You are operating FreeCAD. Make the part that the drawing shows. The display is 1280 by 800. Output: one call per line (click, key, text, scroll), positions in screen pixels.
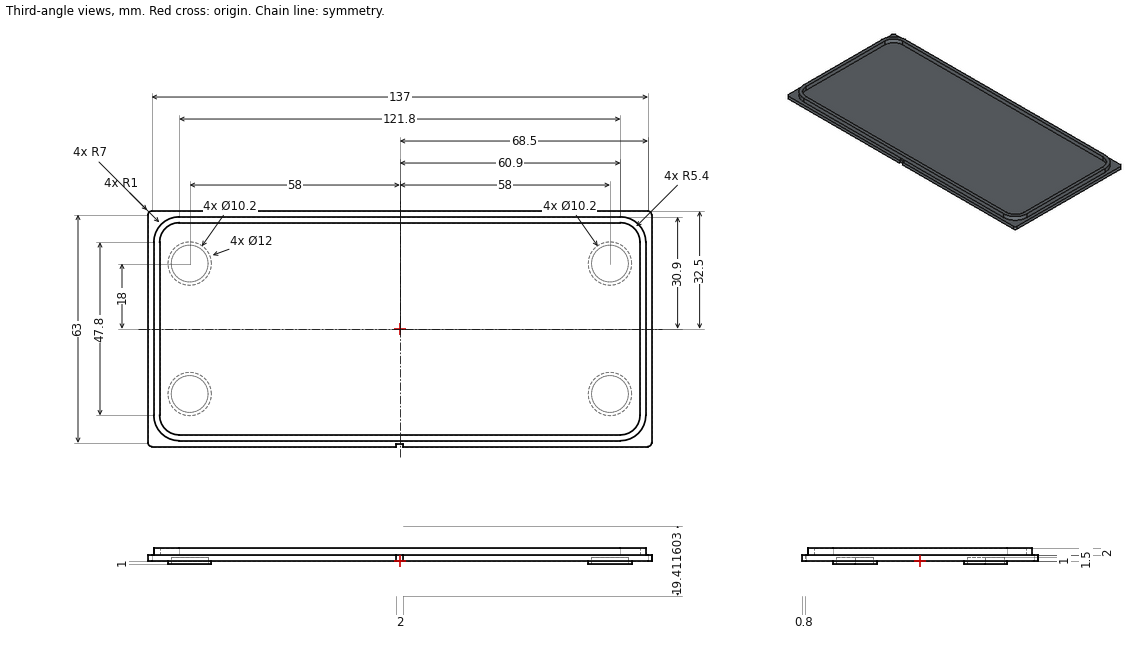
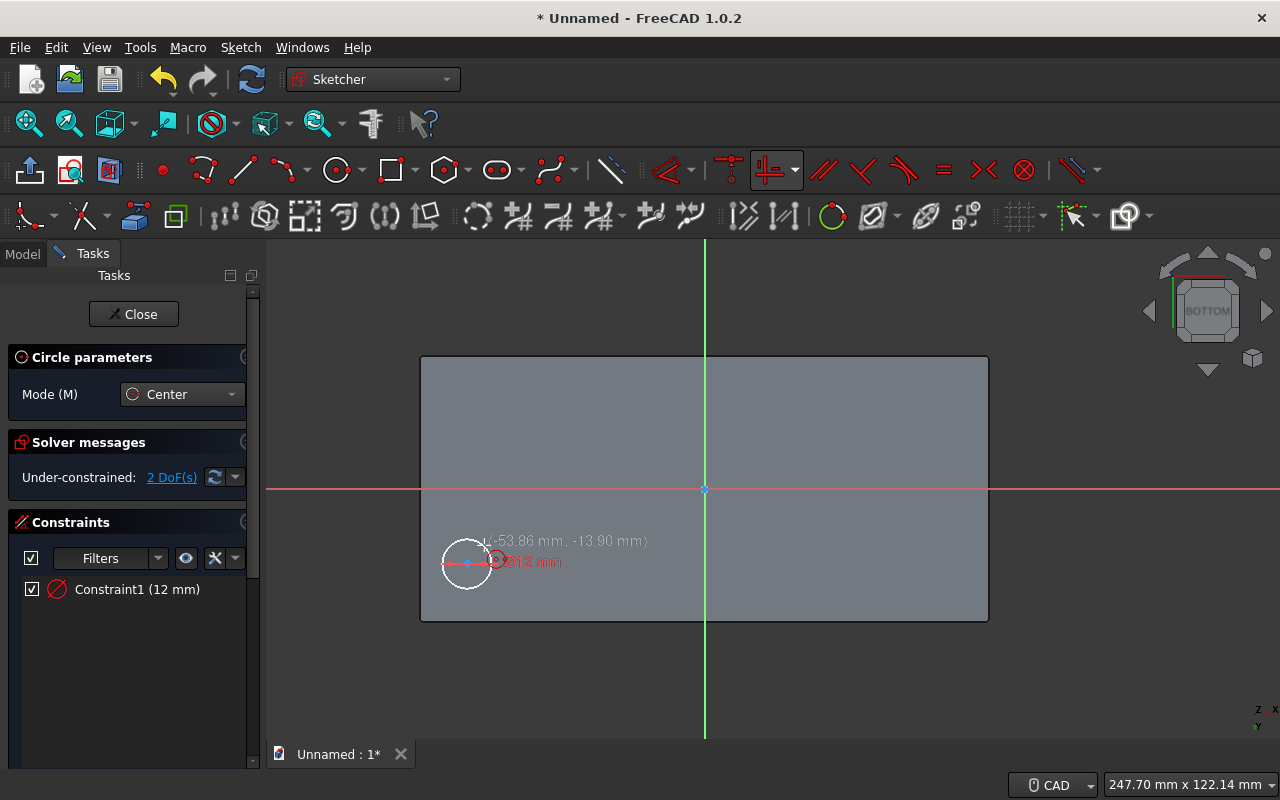
click(942, 563)
move(959, 545)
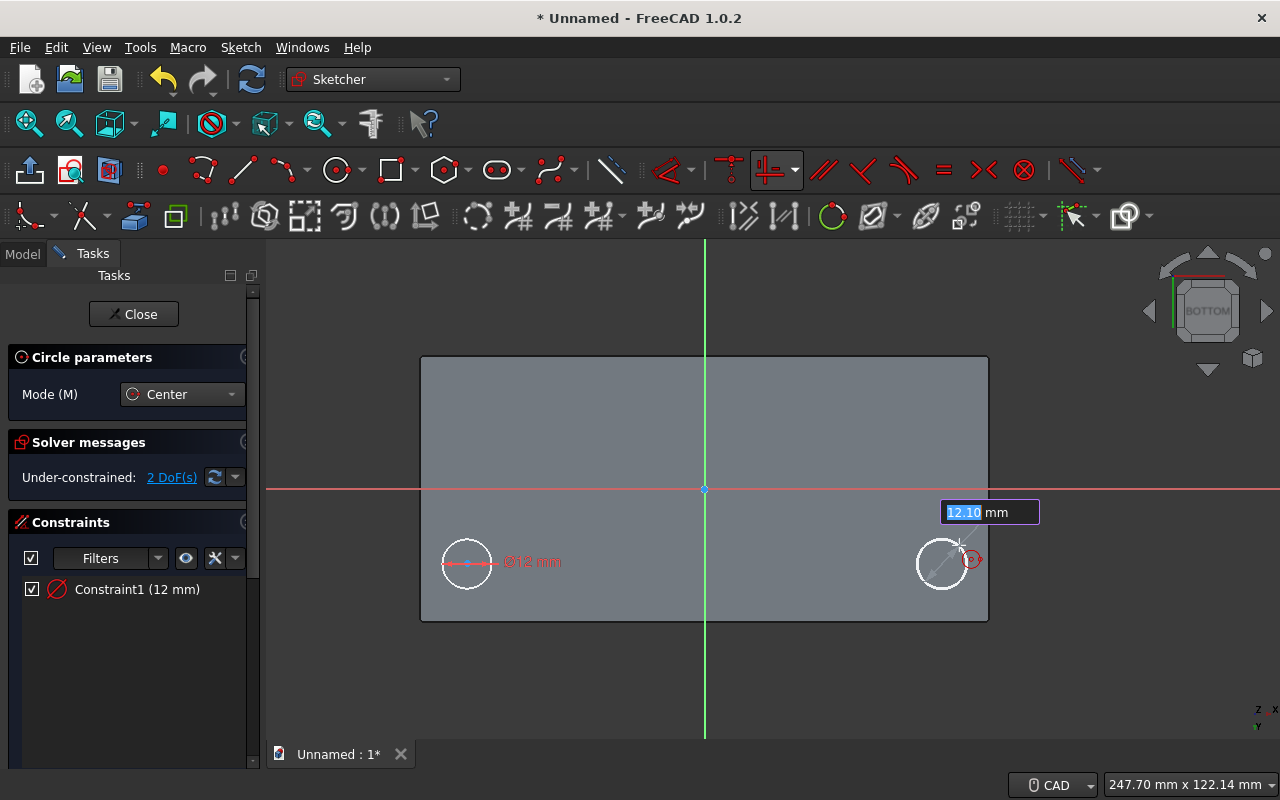
text(12)
key(Return)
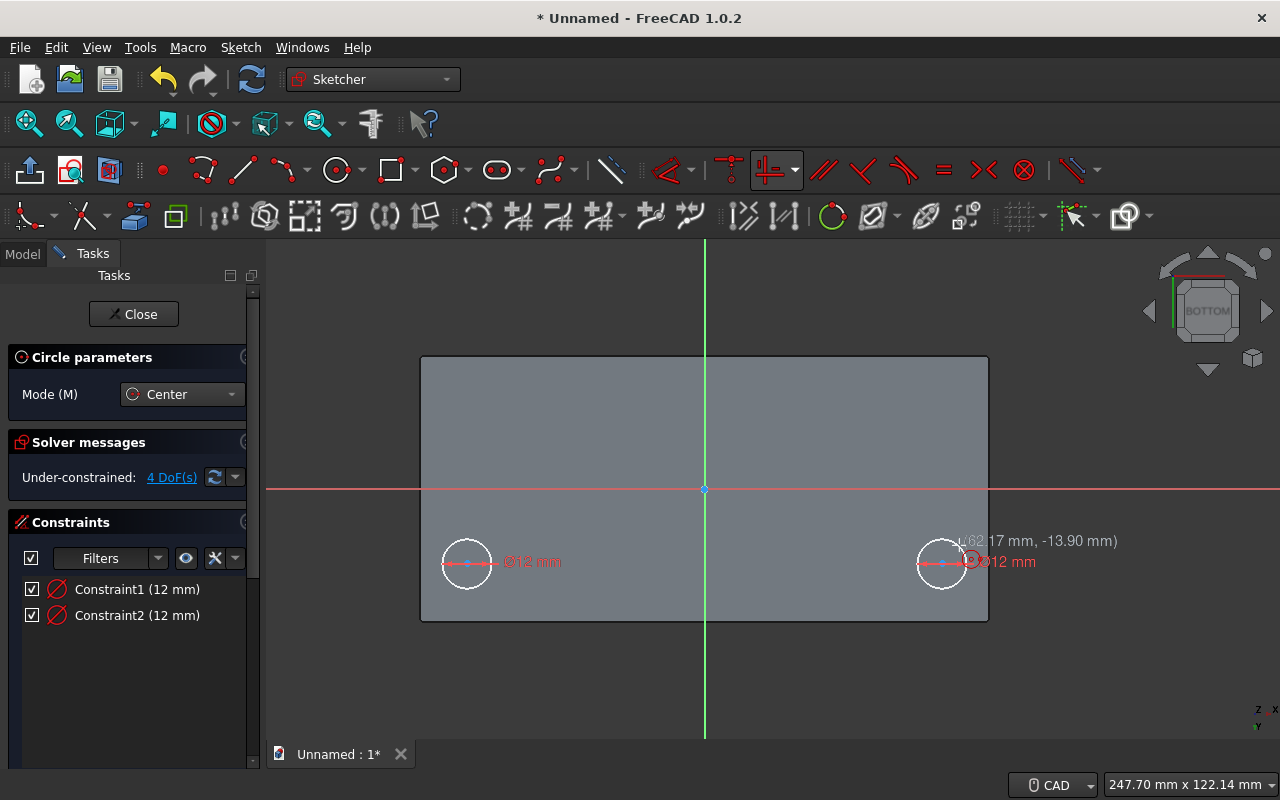
click(467, 415)
move(484, 398)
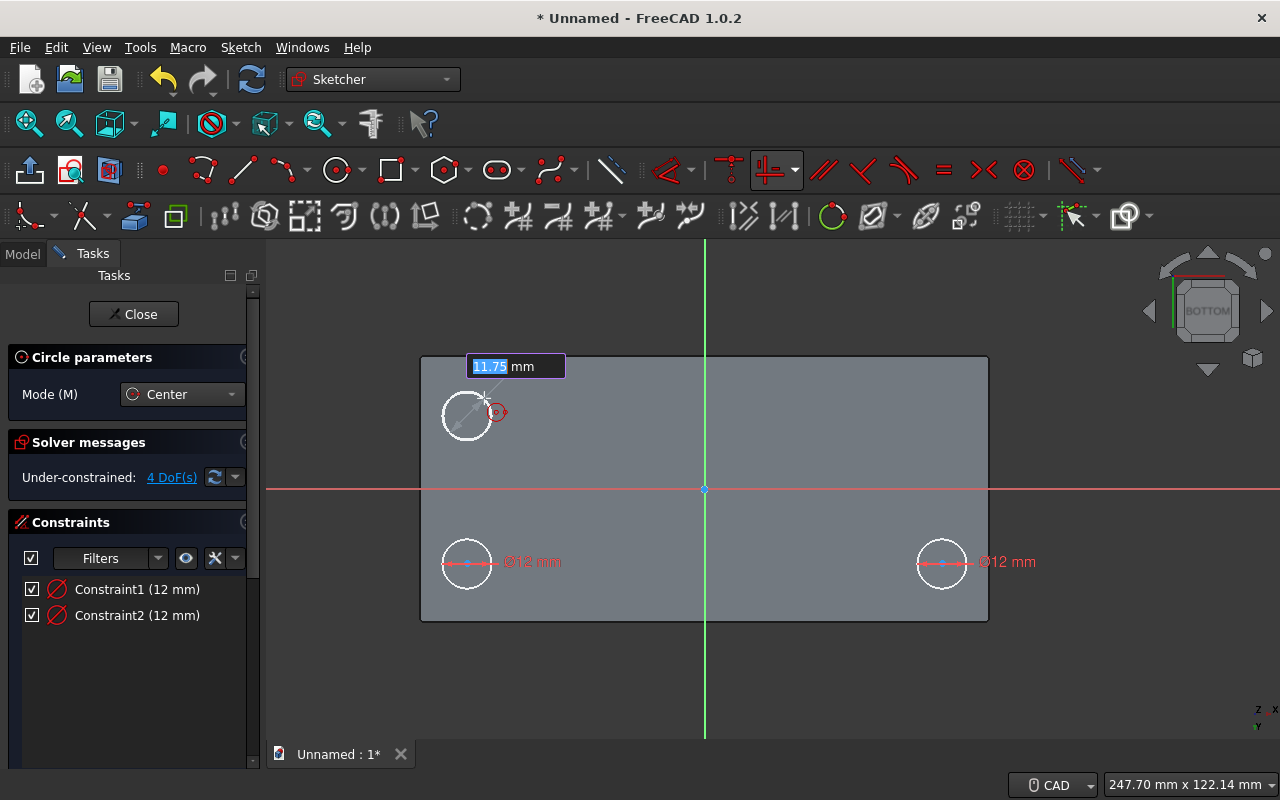
text(12)
key(Return)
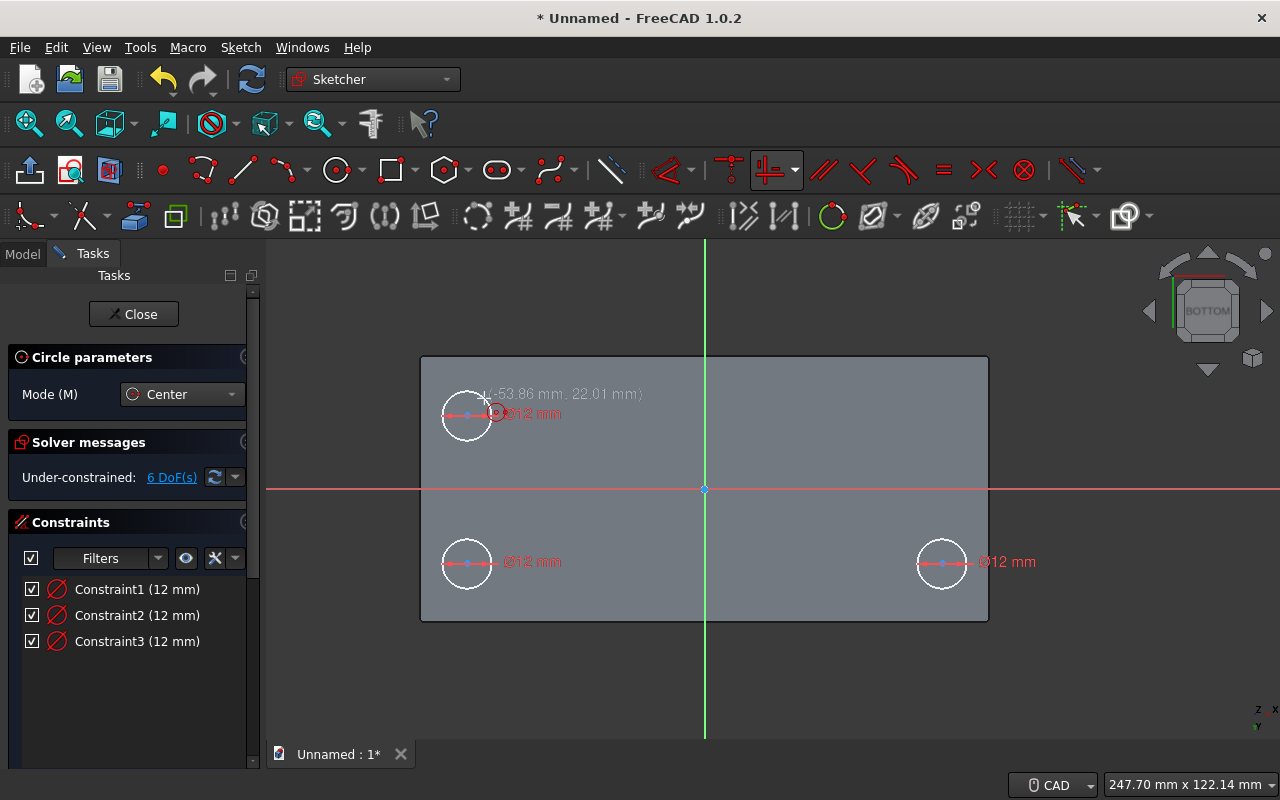
click(942, 415)
move(959, 398)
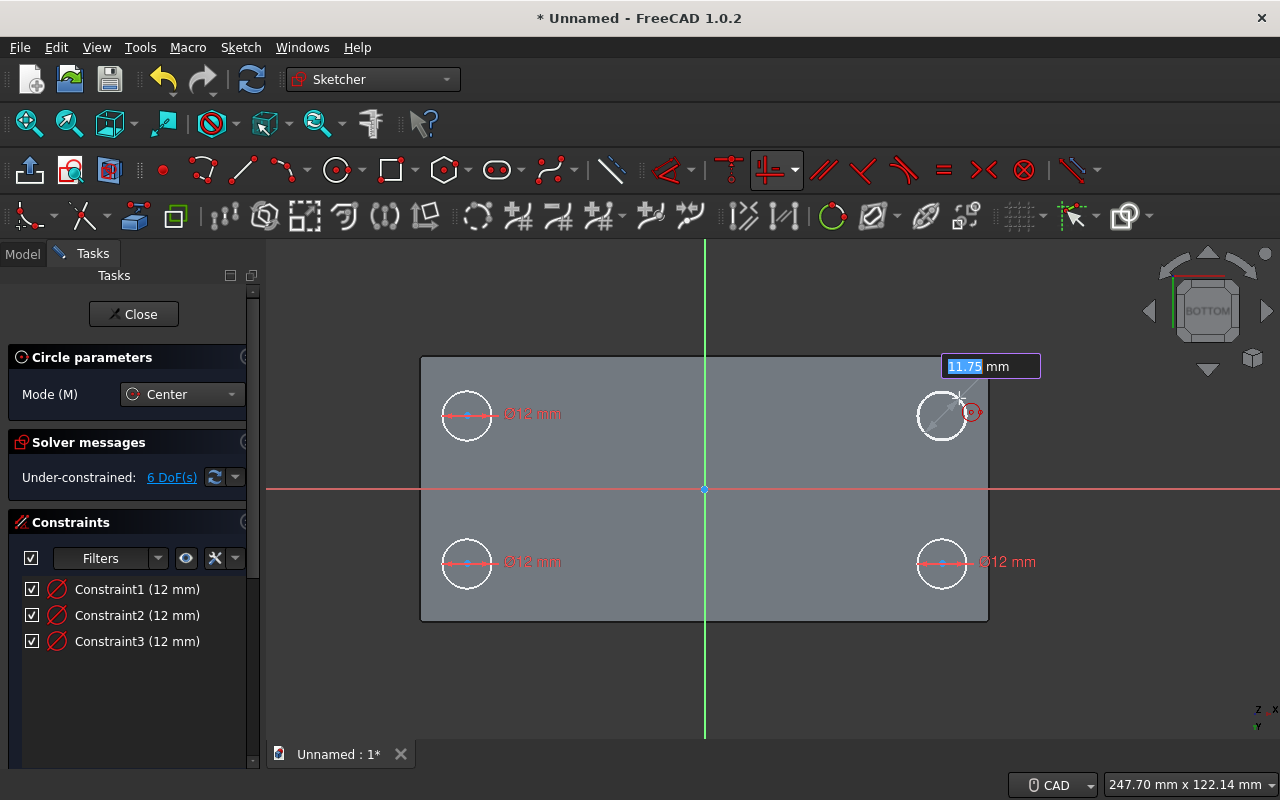
text(12)
key(Return)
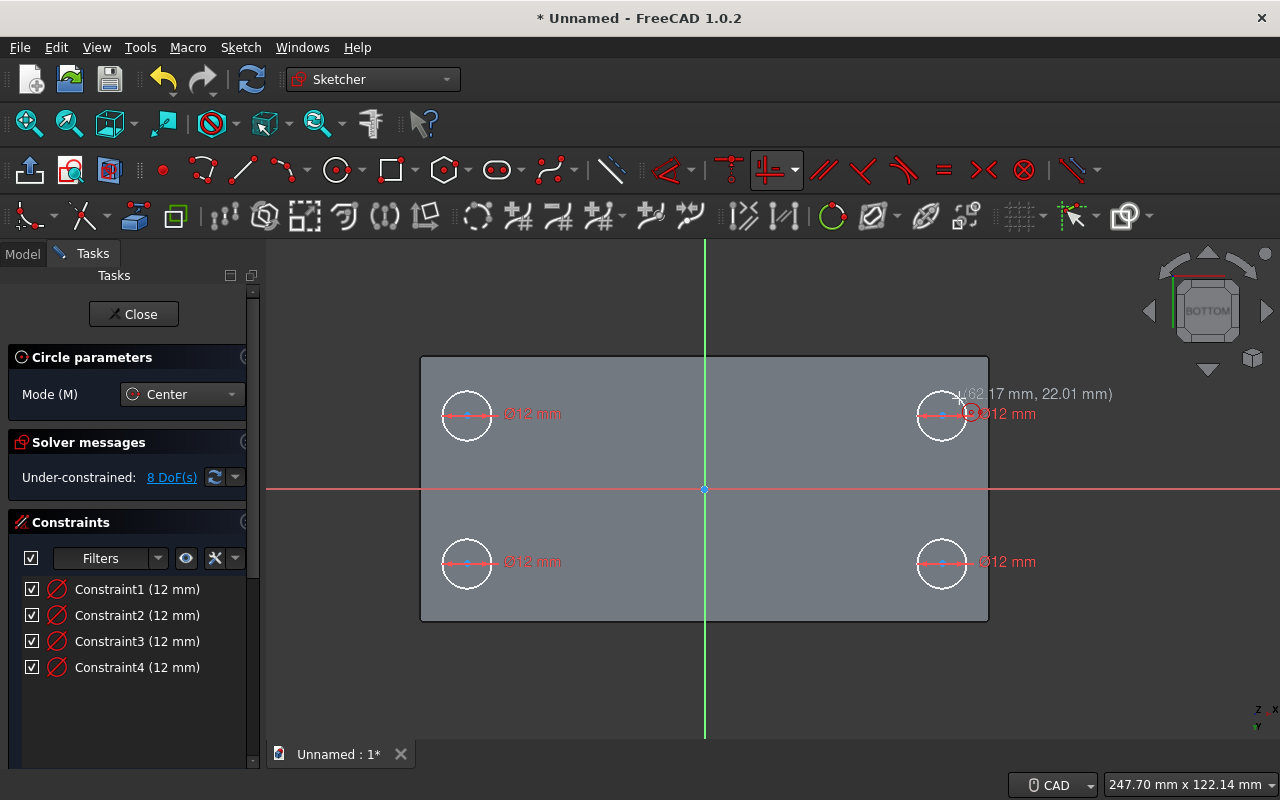
click(467, 564)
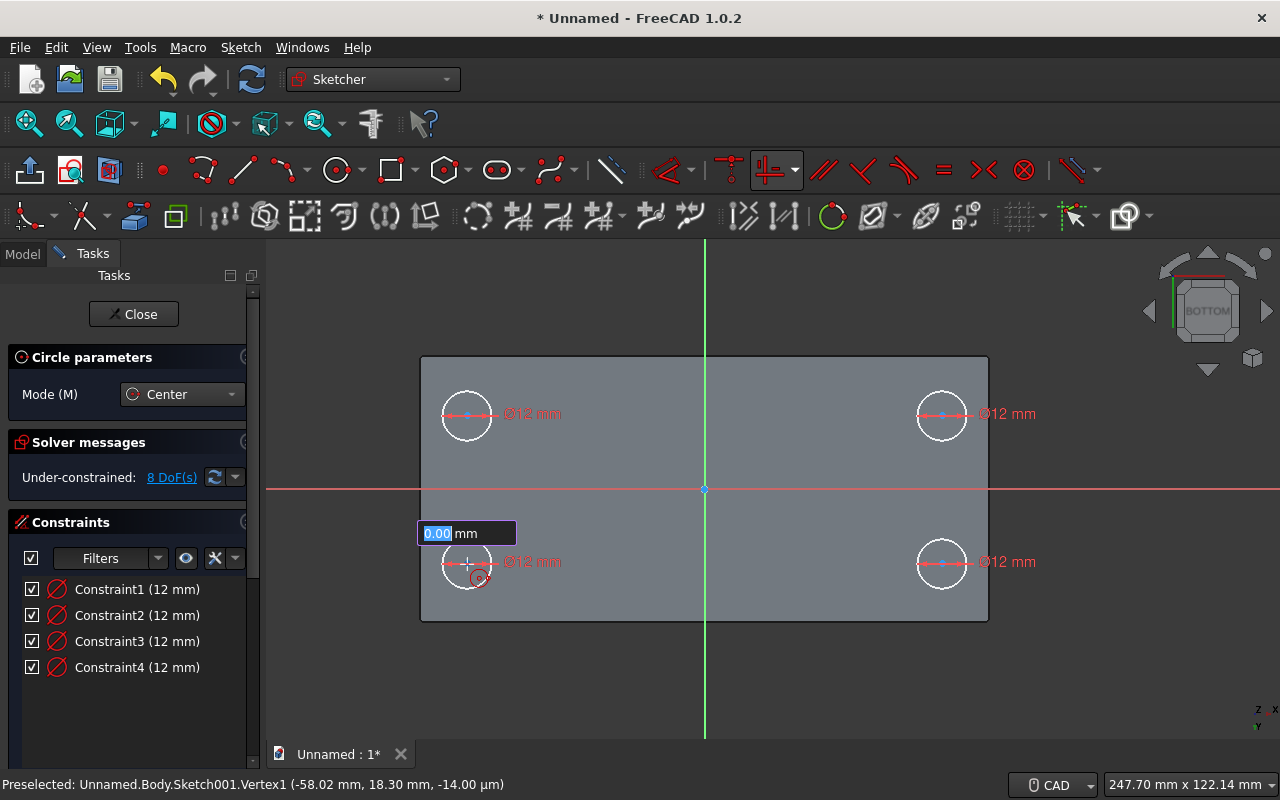
scroll(447, 556, up, 8)
move(449, 552)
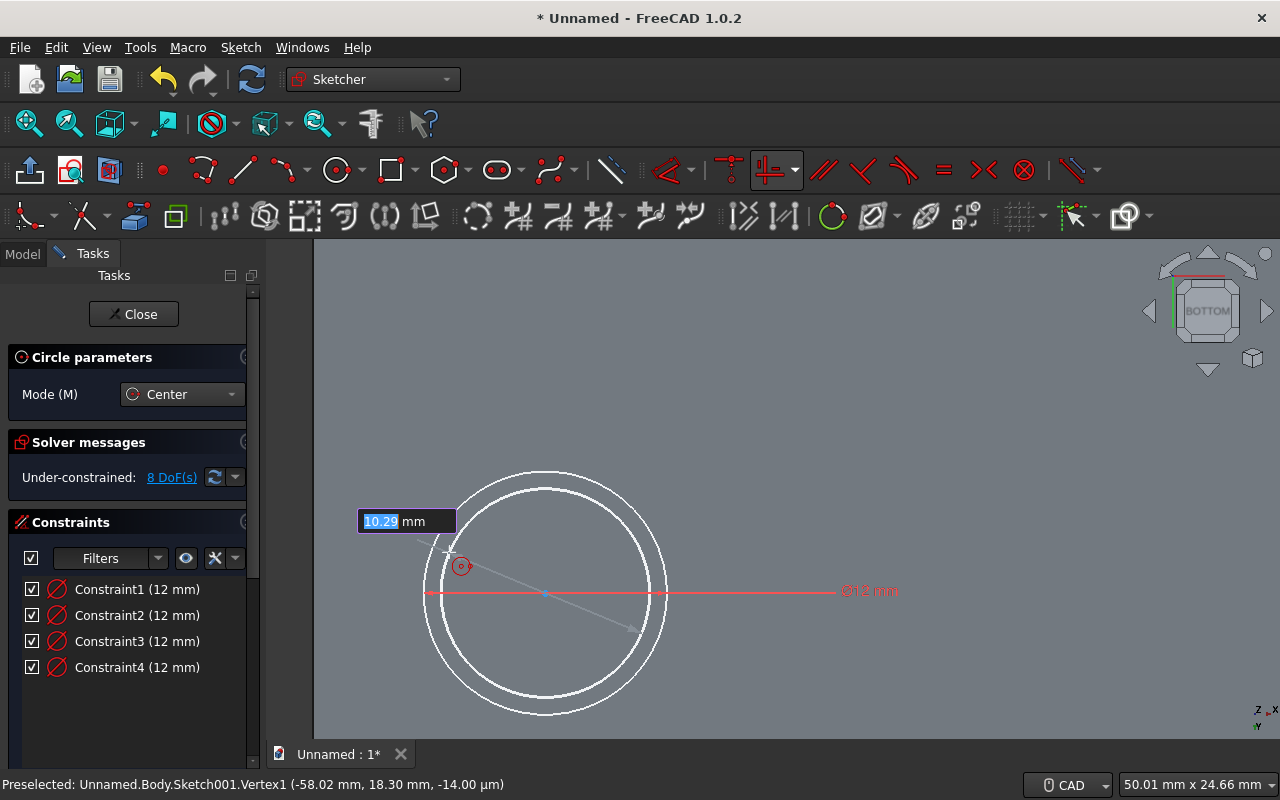
text(10.2)
key(Return)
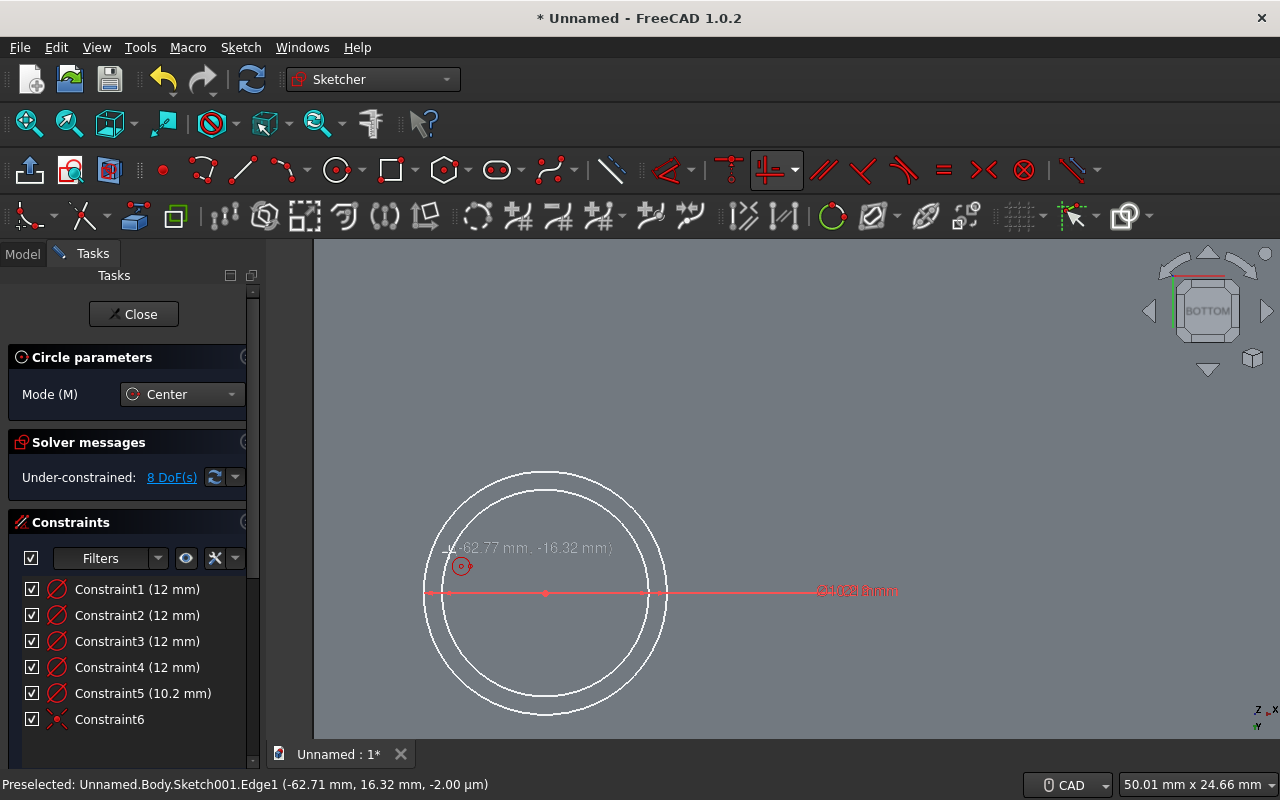
scroll(372, 576, down, 7)